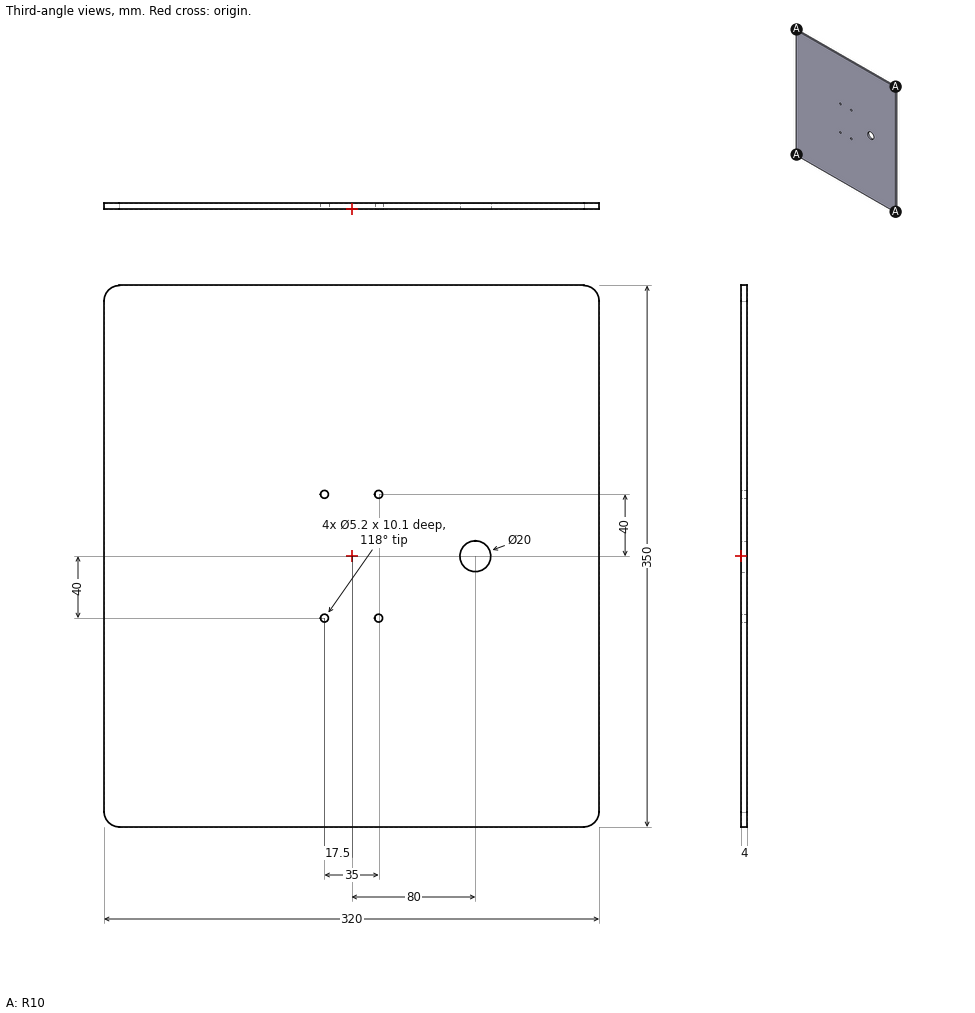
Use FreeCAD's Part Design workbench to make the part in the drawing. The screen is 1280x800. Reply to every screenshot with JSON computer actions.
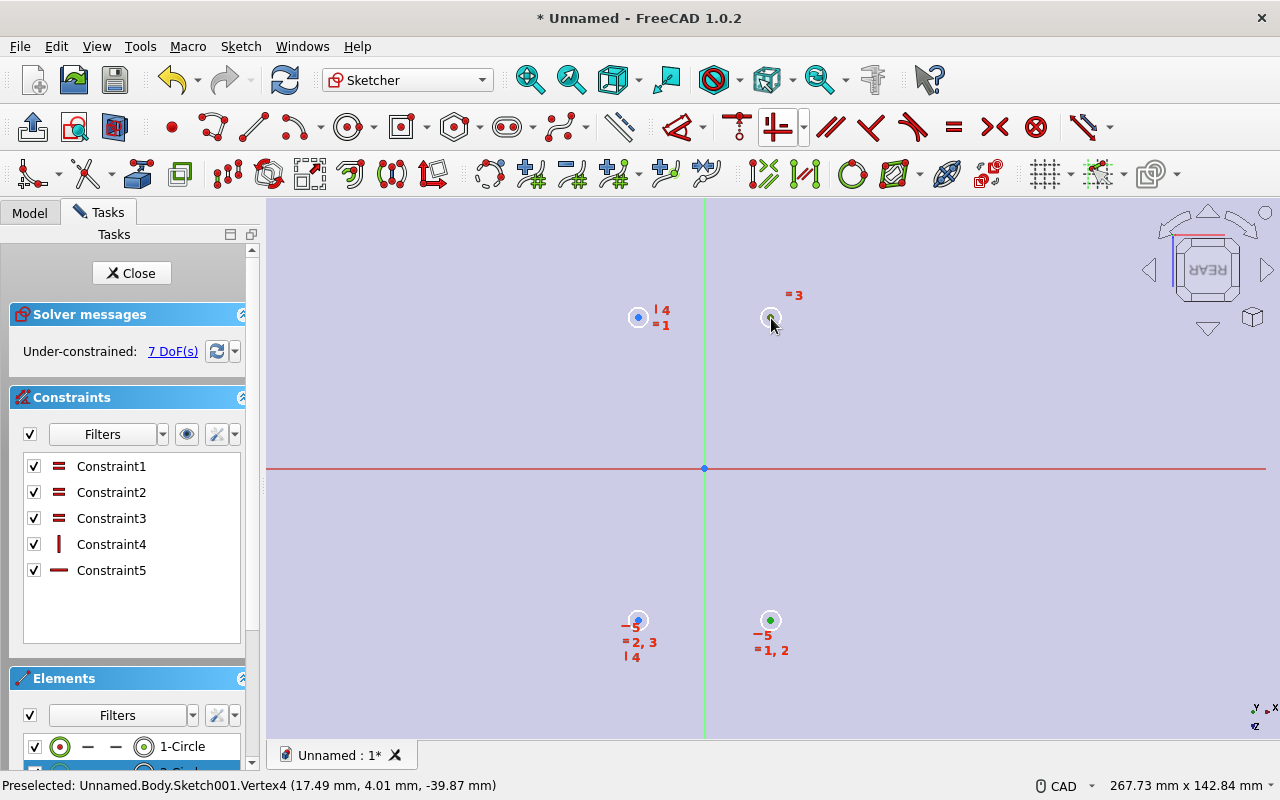
{"action": "left_click", "coordinate": [804, 128]}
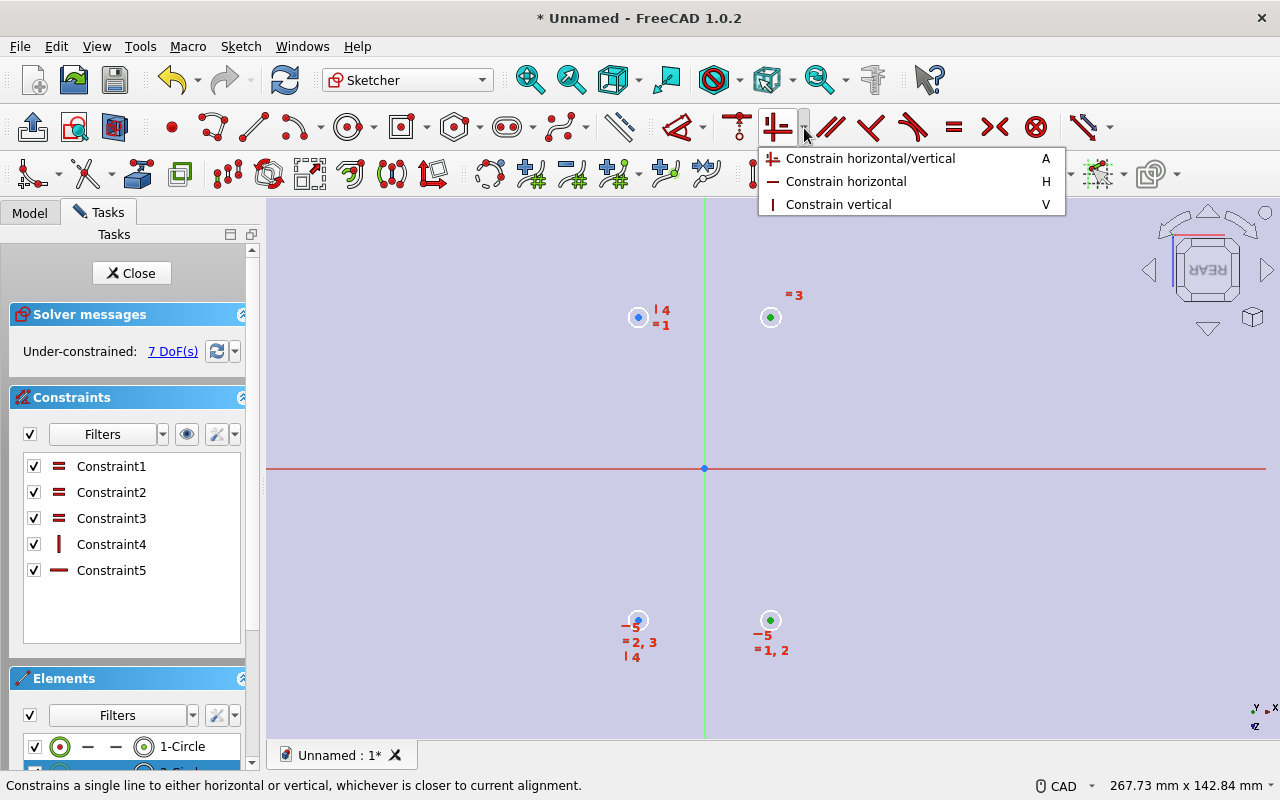
{"action": "left_click", "coordinate": [912, 204]}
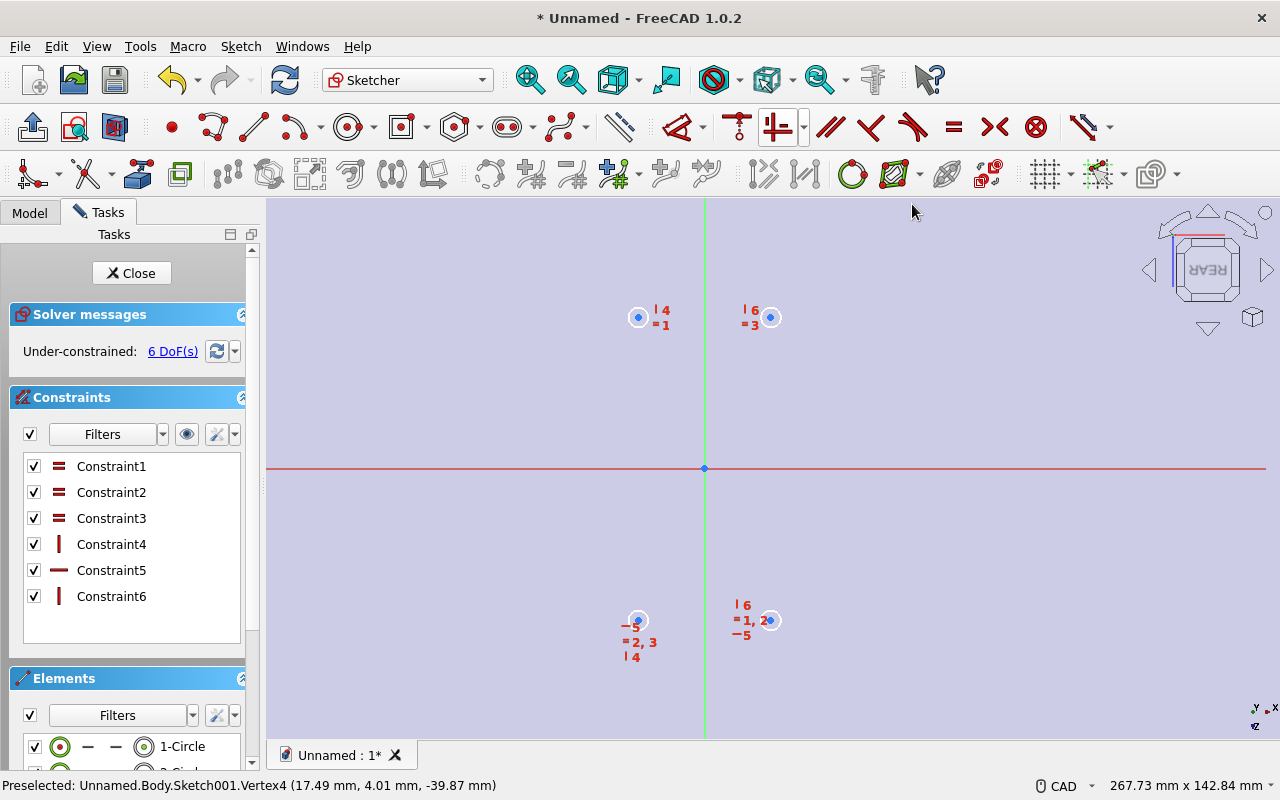
{"action": "left_click", "coordinate": [638, 318]}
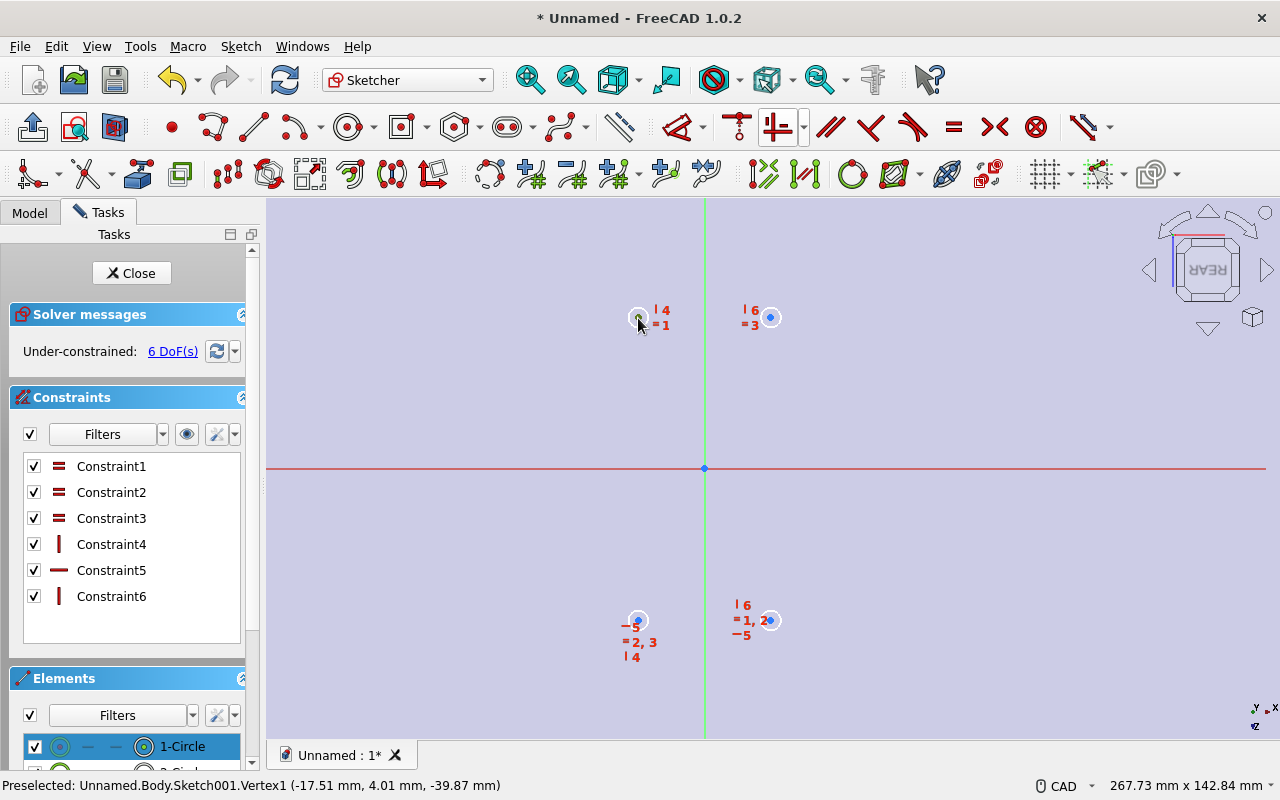
{"action": "left_click", "coordinate": [771, 318]}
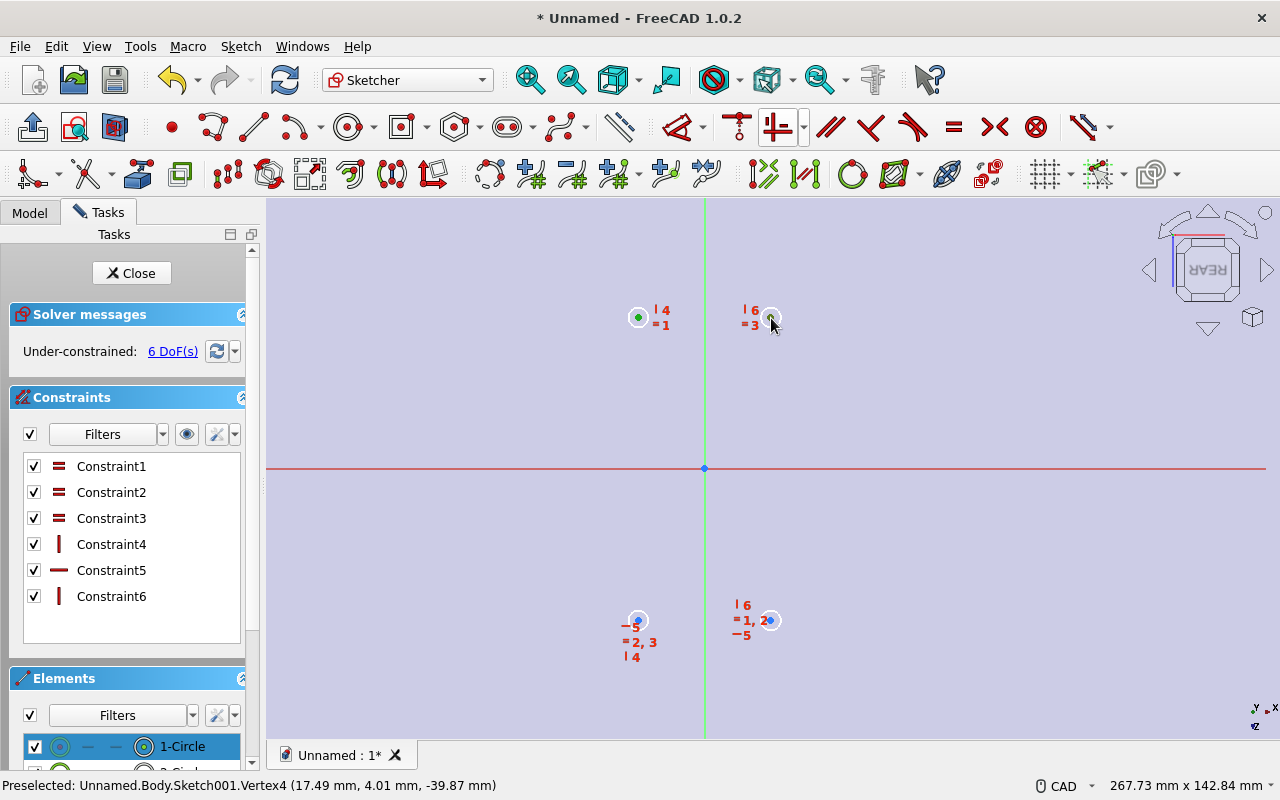
{"action": "key", "text": "h"}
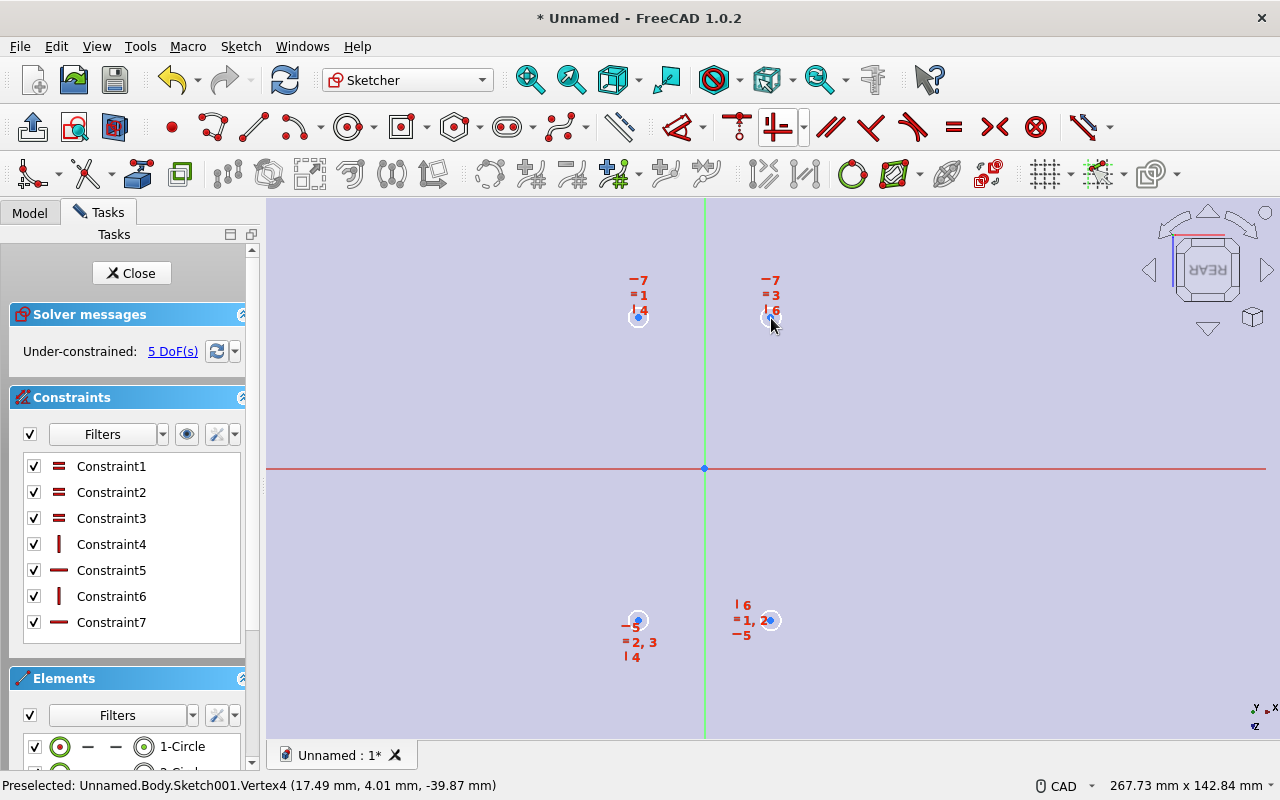
{"action": "left_click", "coordinate": [676, 128]}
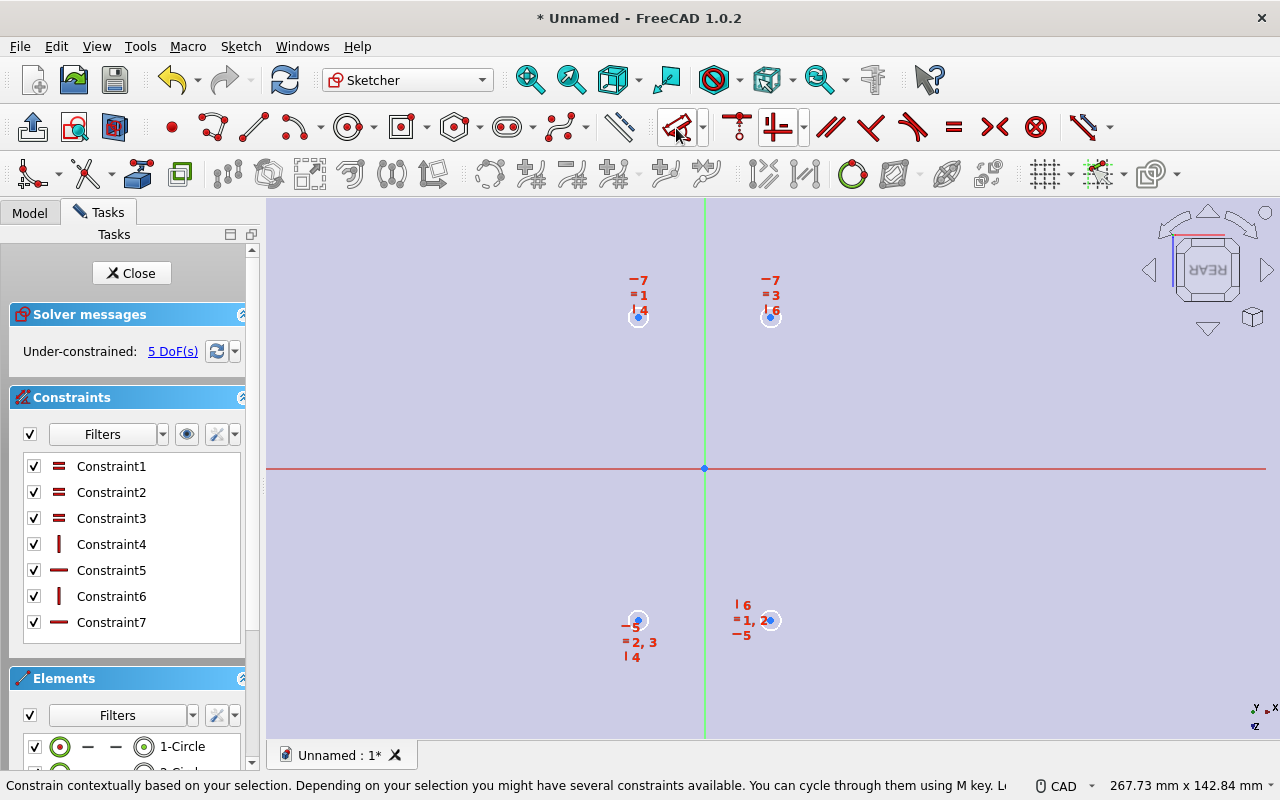
{"action": "scroll", "coordinate": [645, 310], "scroll_direction": "up", "scroll_amount": 4}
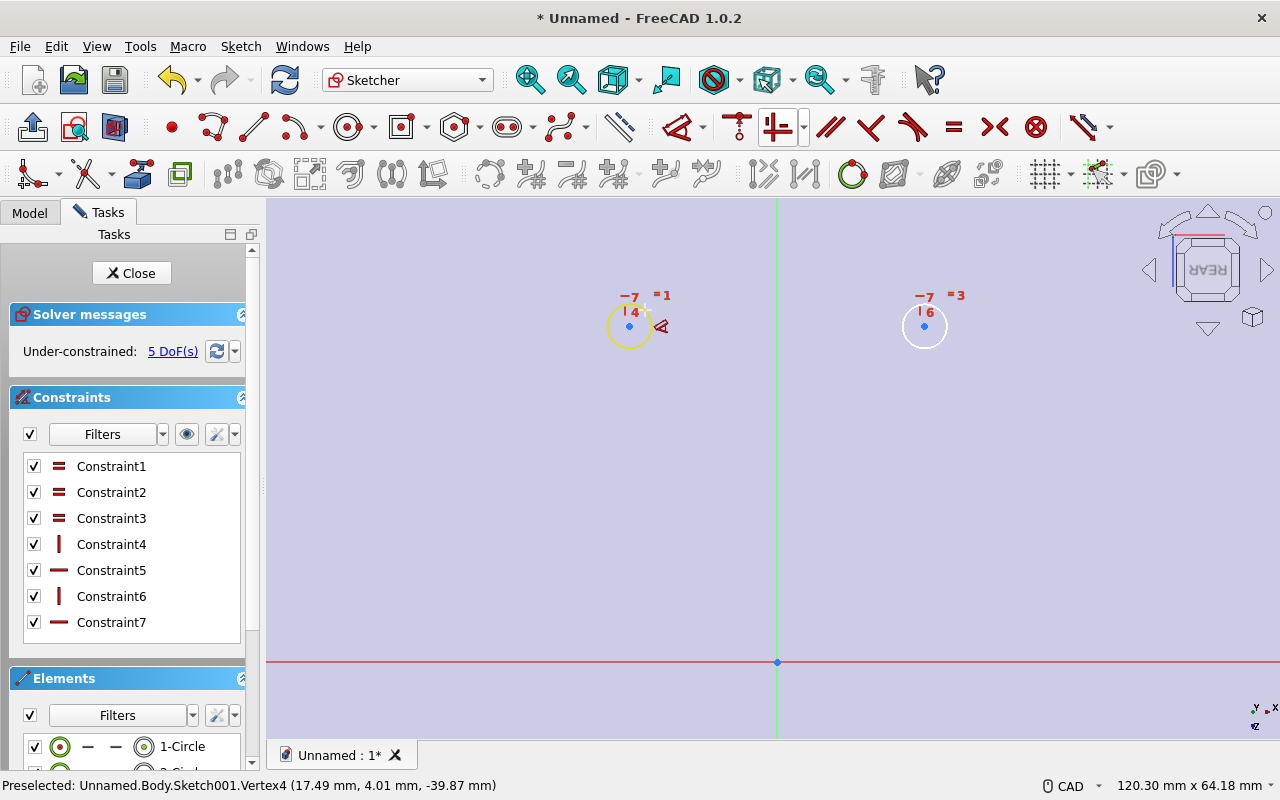
{"action": "left_click", "coordinate": [645, 311]}
{"action": "left_click", "coordinate": [667, 288]}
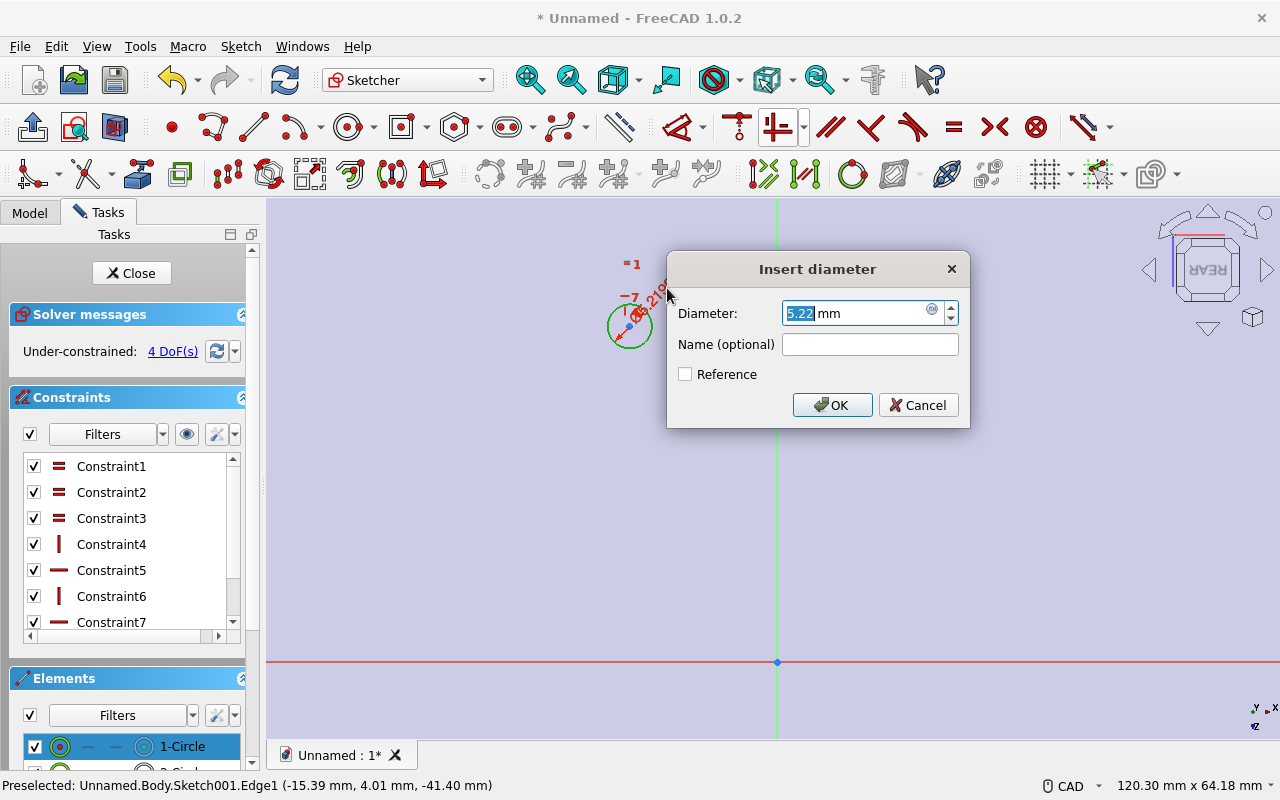
{"action": "type", "text": "5.2"}
{"action": "key", "text": "Return"}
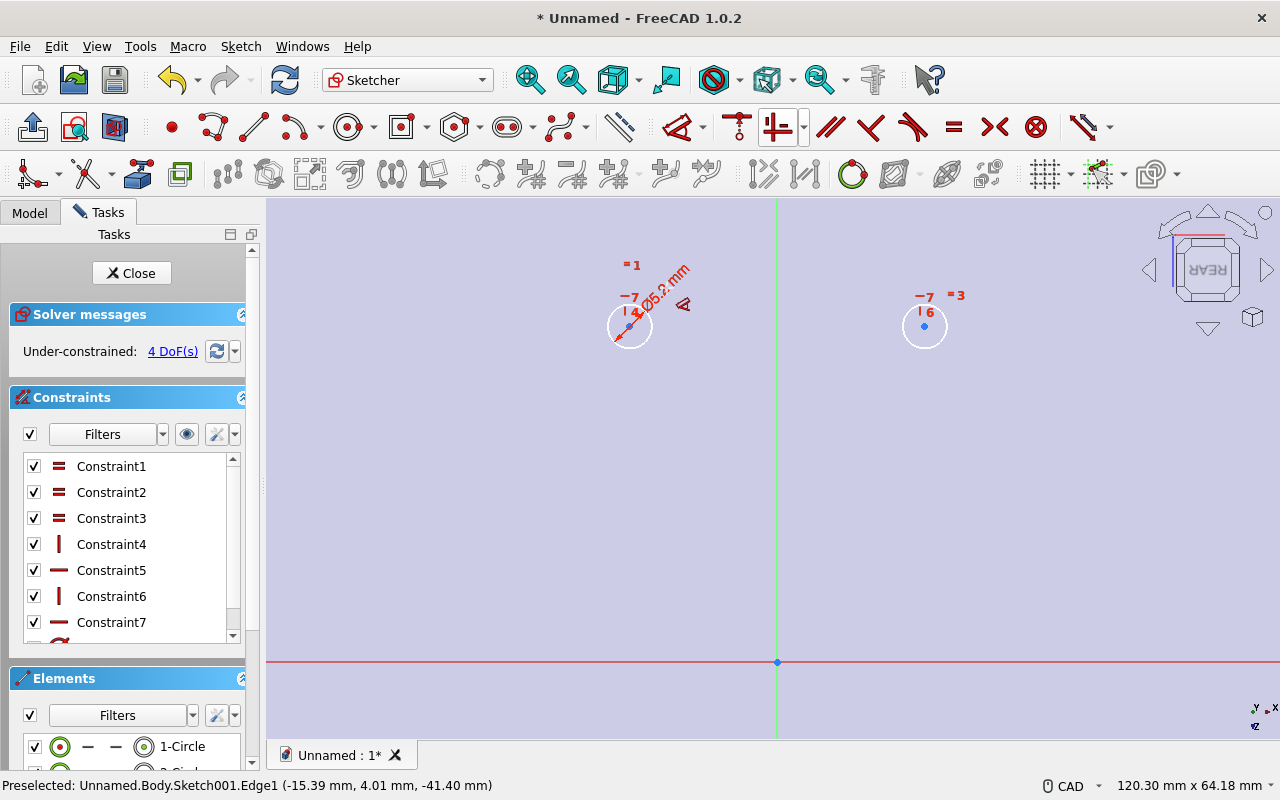
{"action": "left_click", "coordinate": [630, 326]}
{"action": "left_click", "coordinate": [596, 494]}